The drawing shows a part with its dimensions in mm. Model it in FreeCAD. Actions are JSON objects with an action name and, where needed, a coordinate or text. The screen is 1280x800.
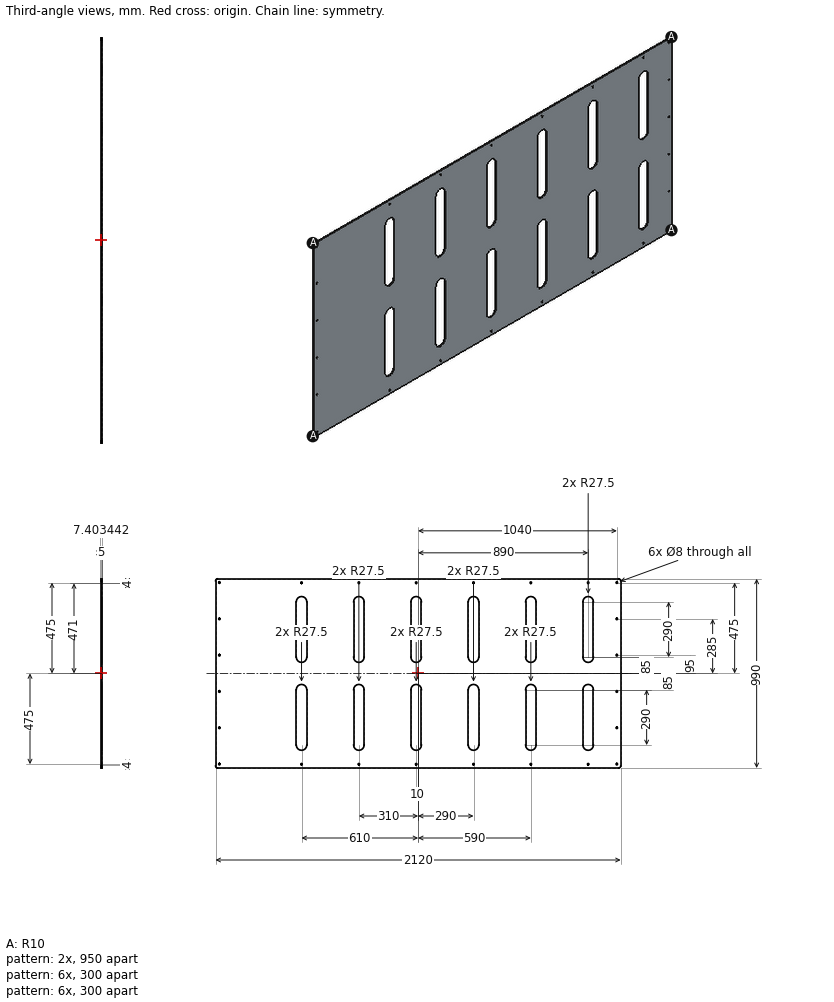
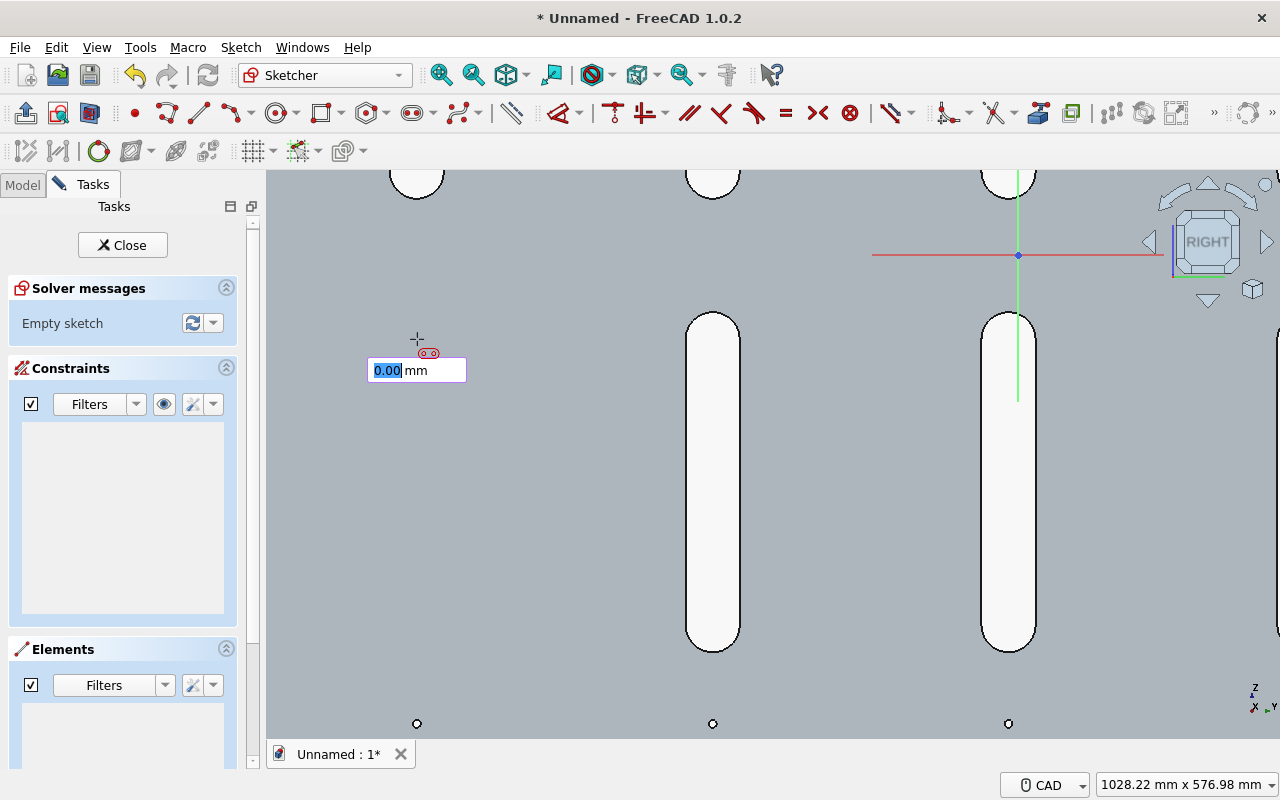
{"action": "left_click", "coordinate": [444, 482]}
{"action": "key", "text": "Escape"}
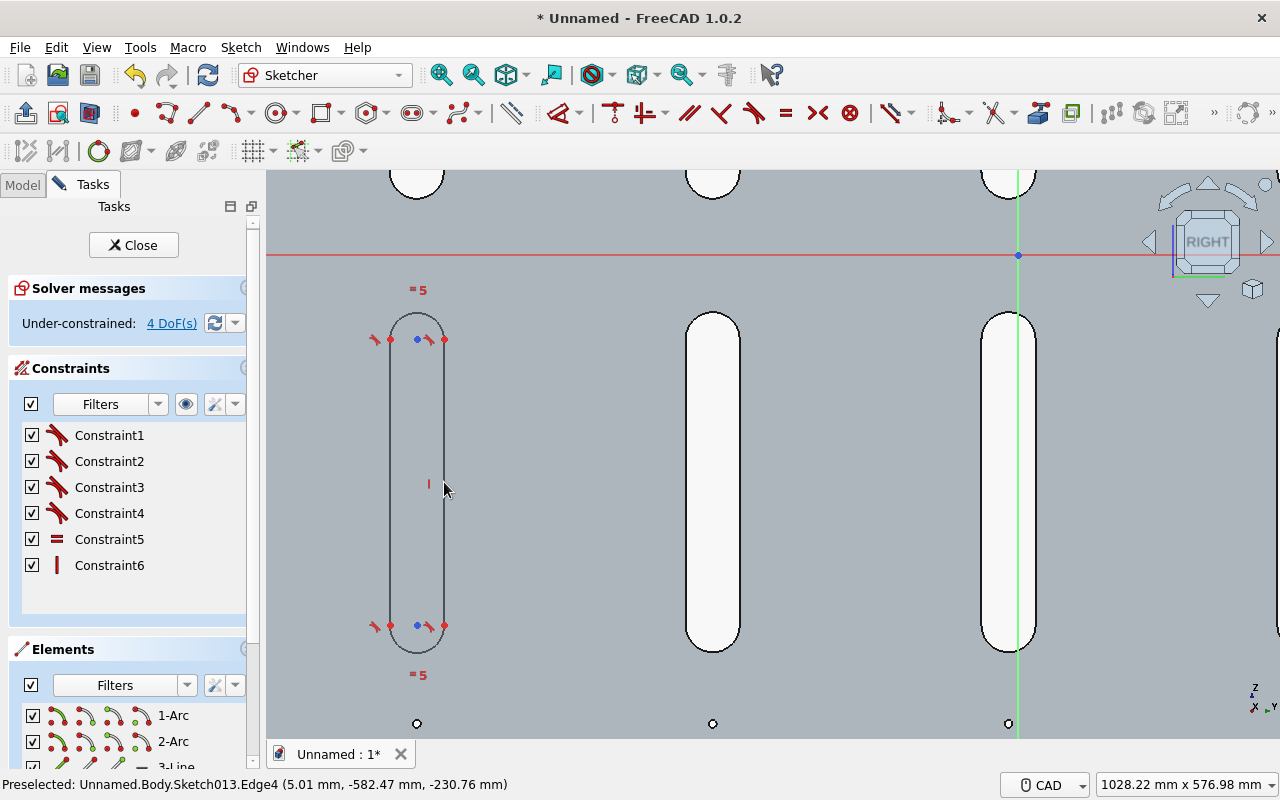
{"action": "left_click", "coordinate": [558, 114]}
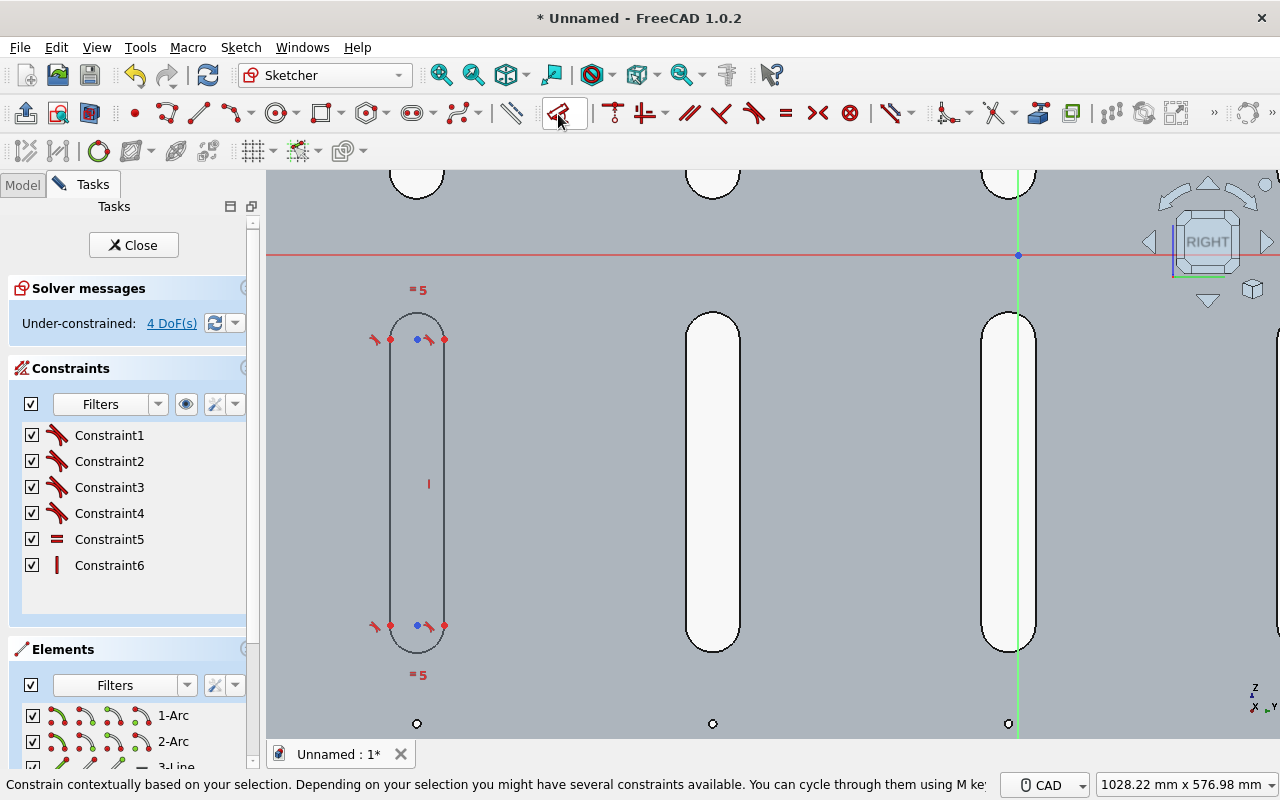
{"action": "scroll", "coordinate": [401, 648], "scroll_direction": "up", "scroll_amount": 2}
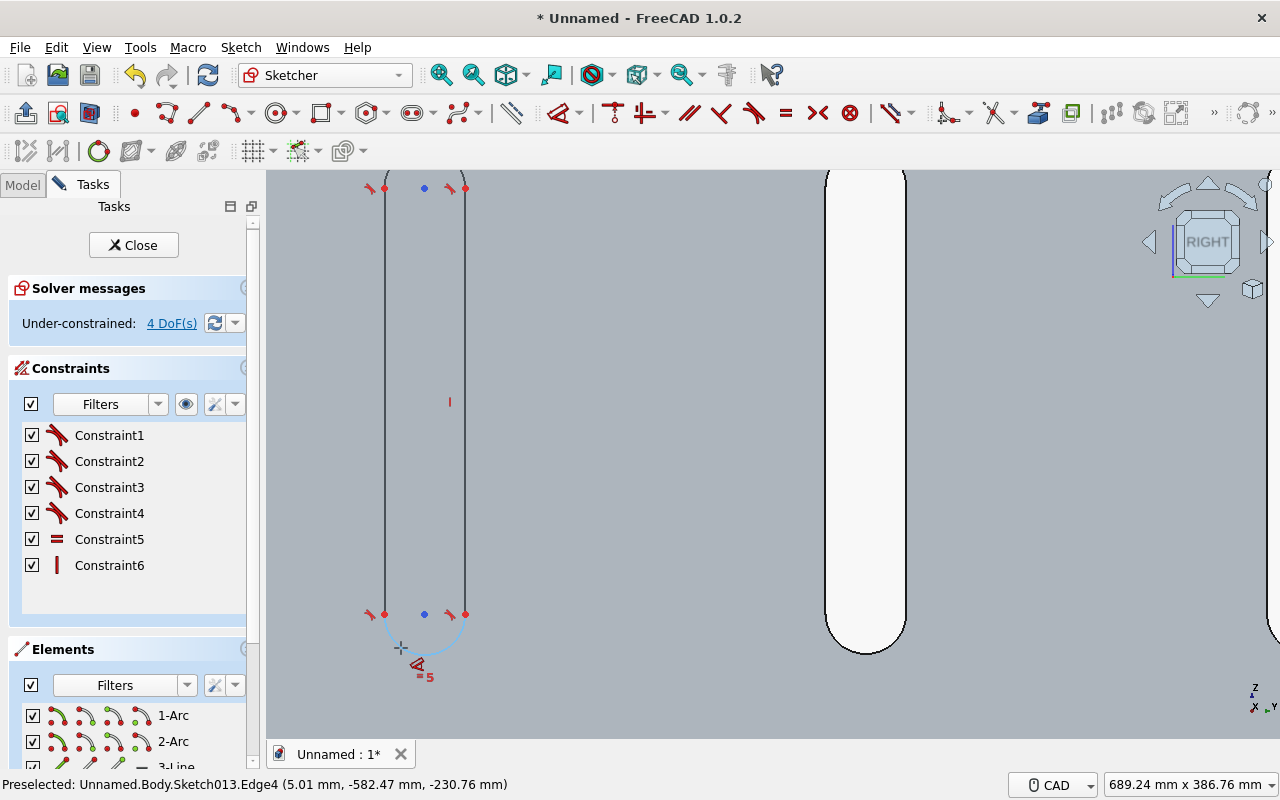
{"action": "left_click", "coordinate": [401, 647]}
{"action": "left_click", "coordinate": [382, 673]}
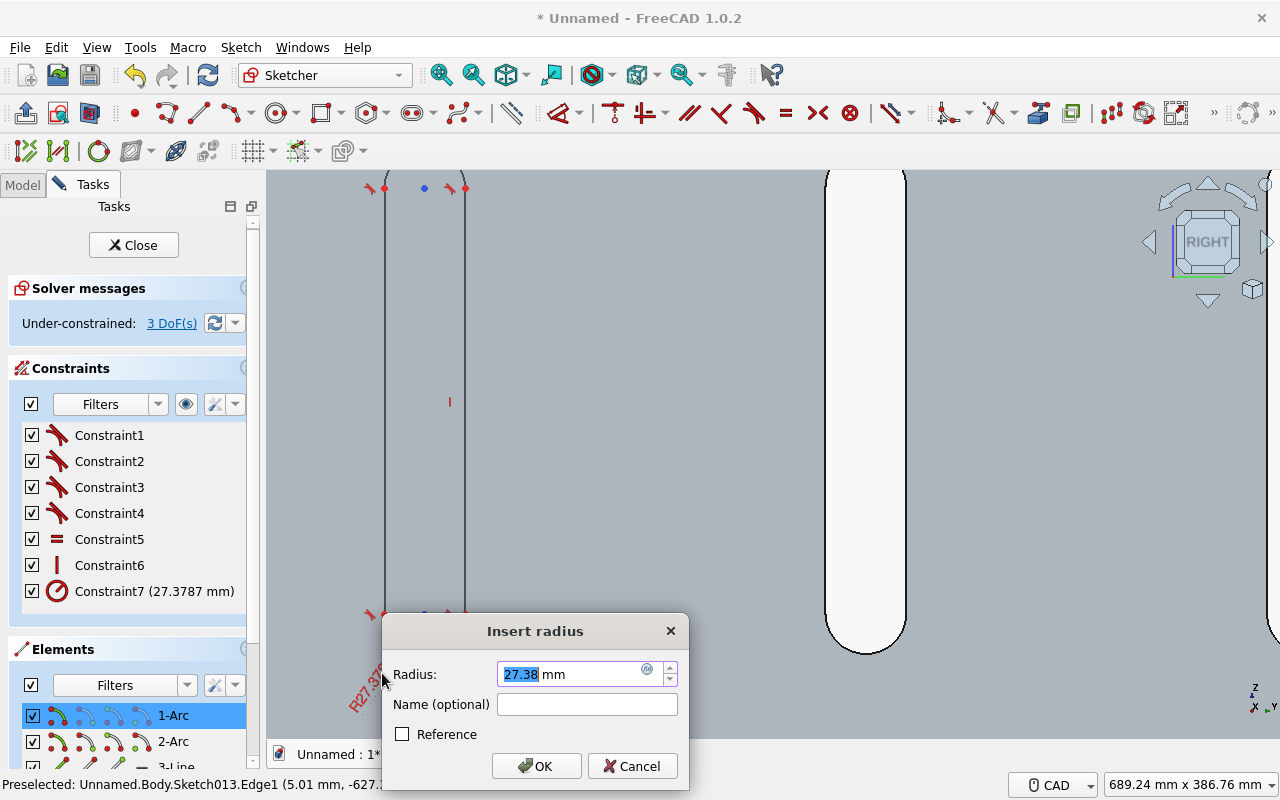
{"action": "type", "text": "27.5"}
{"action": "key", "text": "Return"}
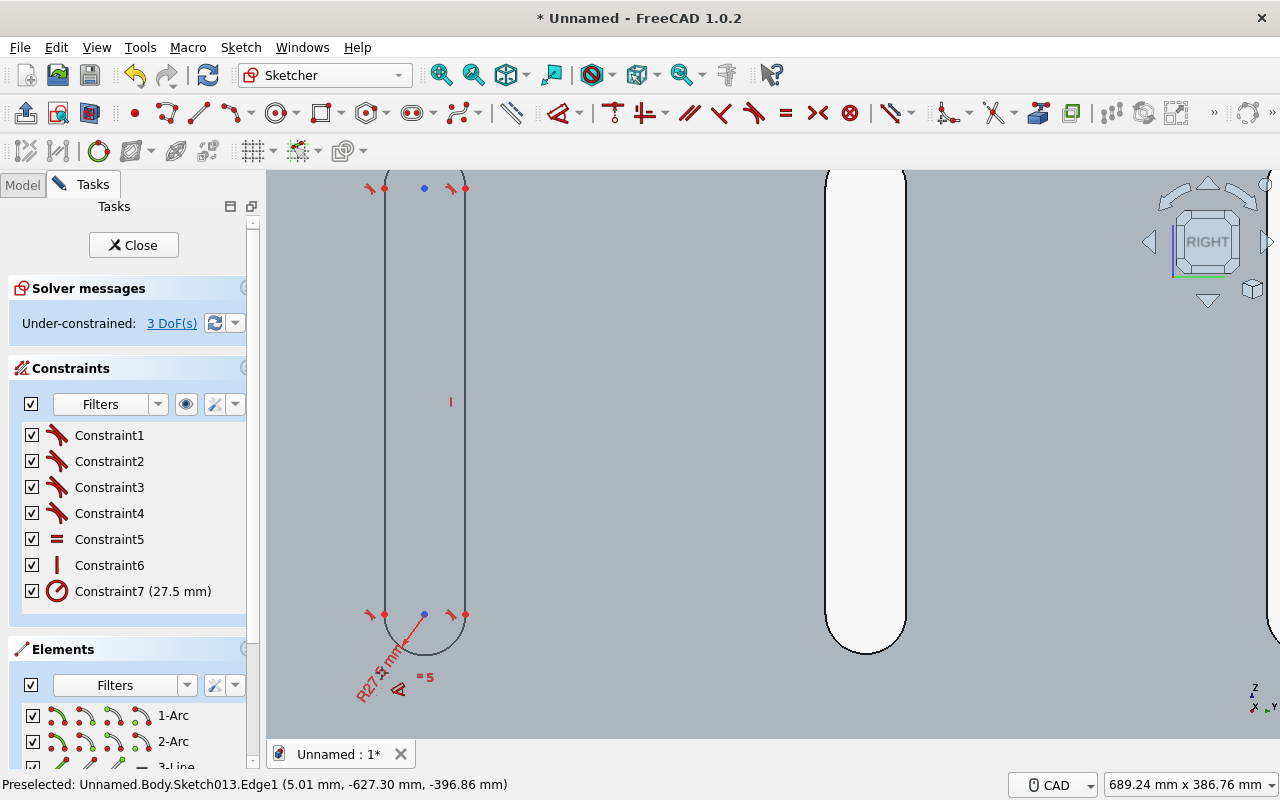
{"action": "left_click", "coordinate": [385, 487]}
{"action": "left_click", "coordinate": [351, 406]}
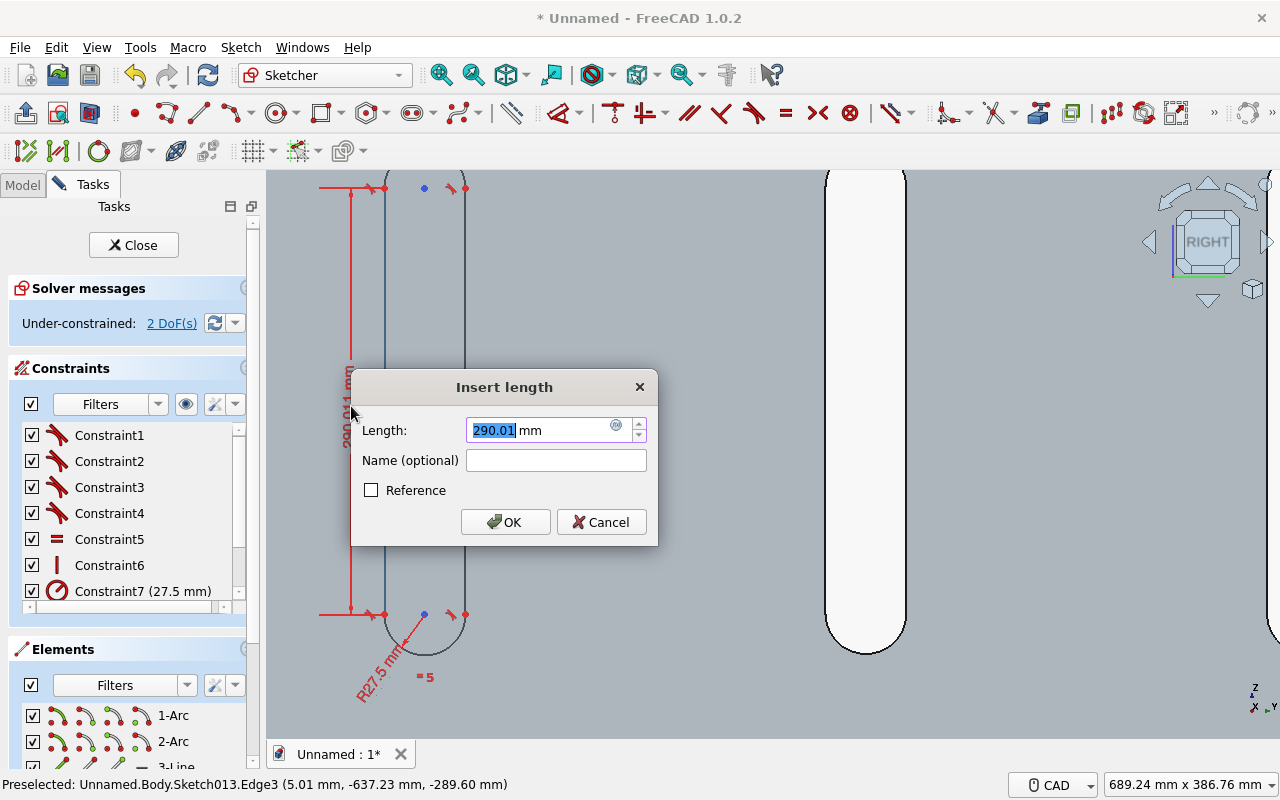
{"action": "type", "text": "290"}
{"action": "key", "text": "Return"}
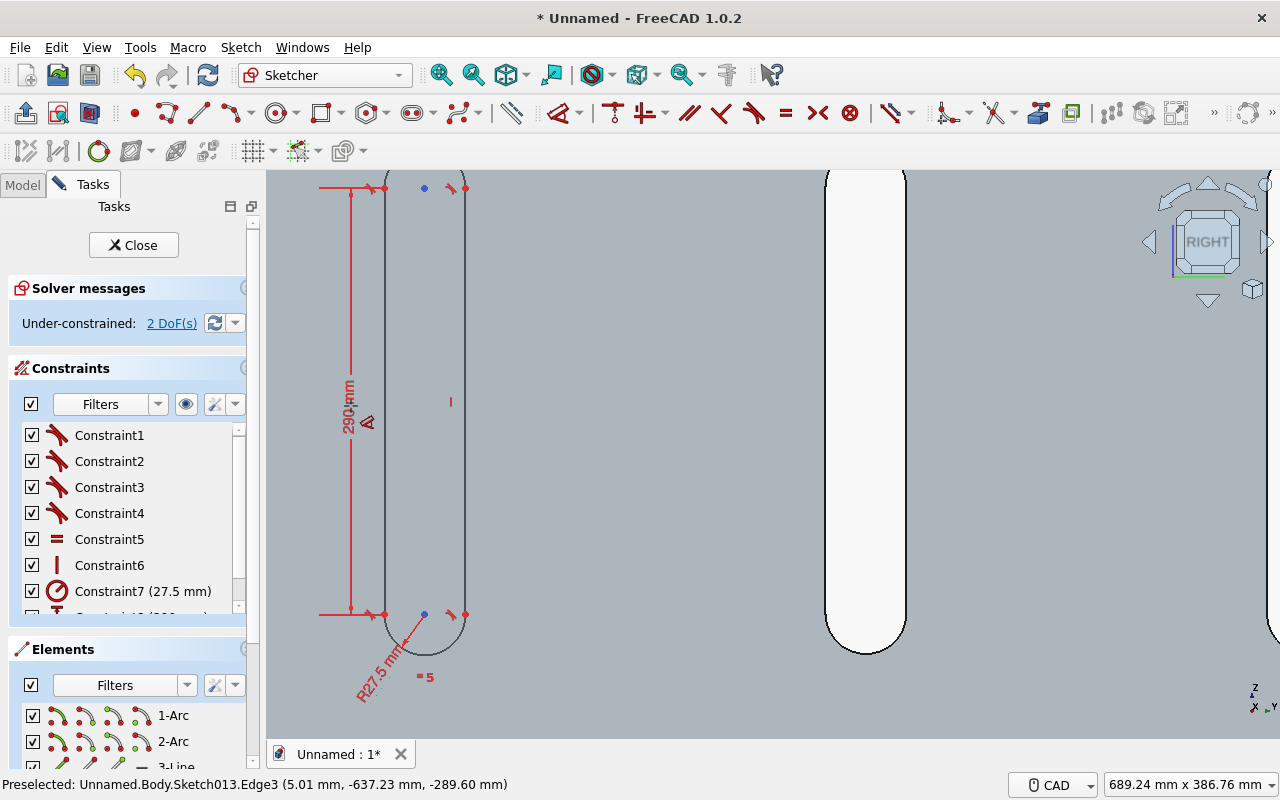
{"action": "scroll", "coordinate": [402, 651], "scroll_direction": "down", "scroll_amount": 2}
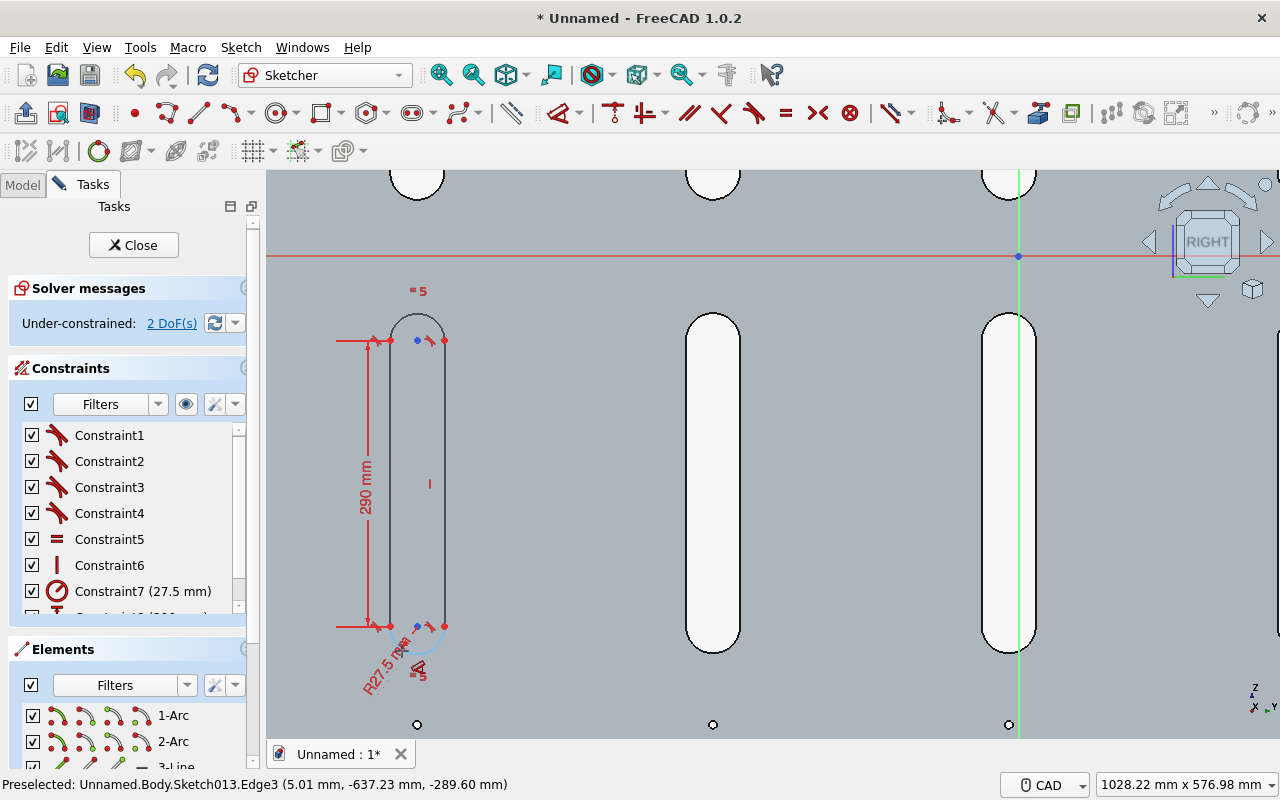
{"action": "left_click", "coordinate": [445, 341]}
{"action": "left_click", "coordinate": [1053, 299]}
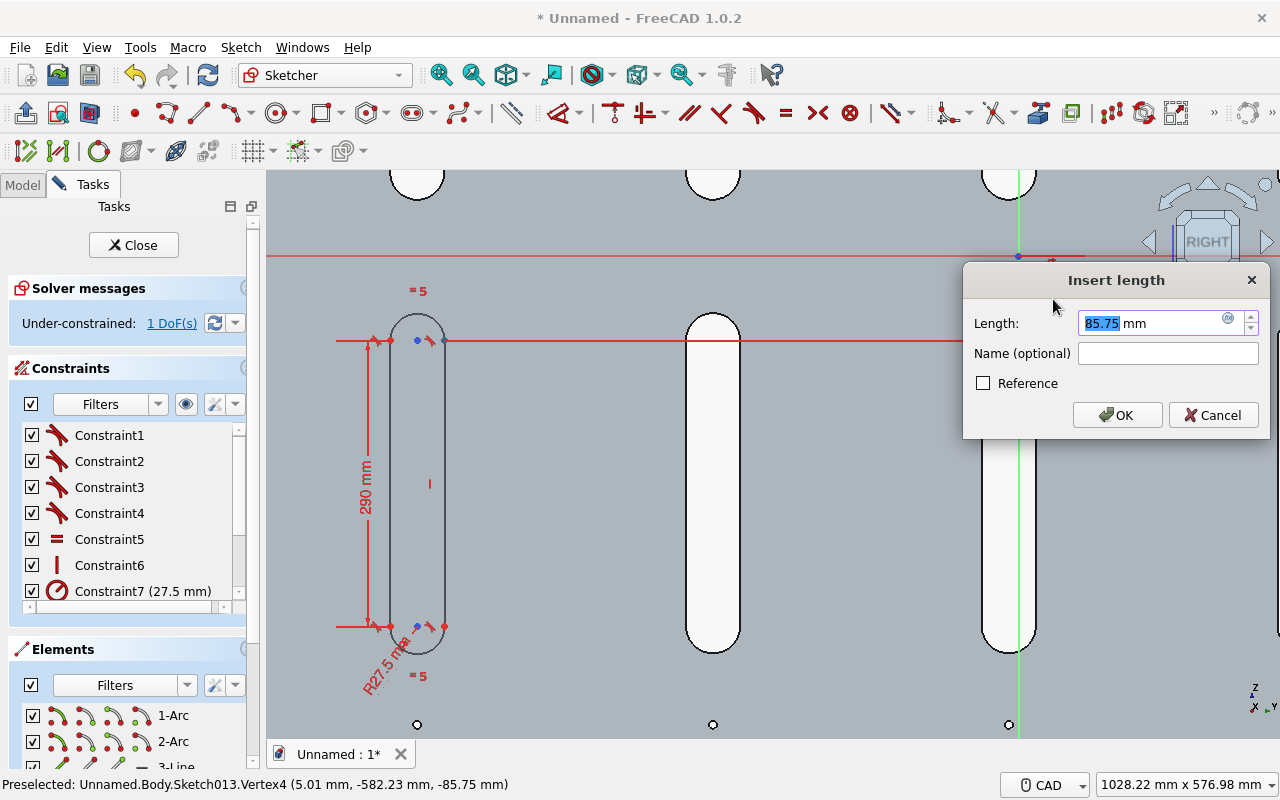
{"action": "type", "text": "85"}
{"action": "key", "text": "Return"}